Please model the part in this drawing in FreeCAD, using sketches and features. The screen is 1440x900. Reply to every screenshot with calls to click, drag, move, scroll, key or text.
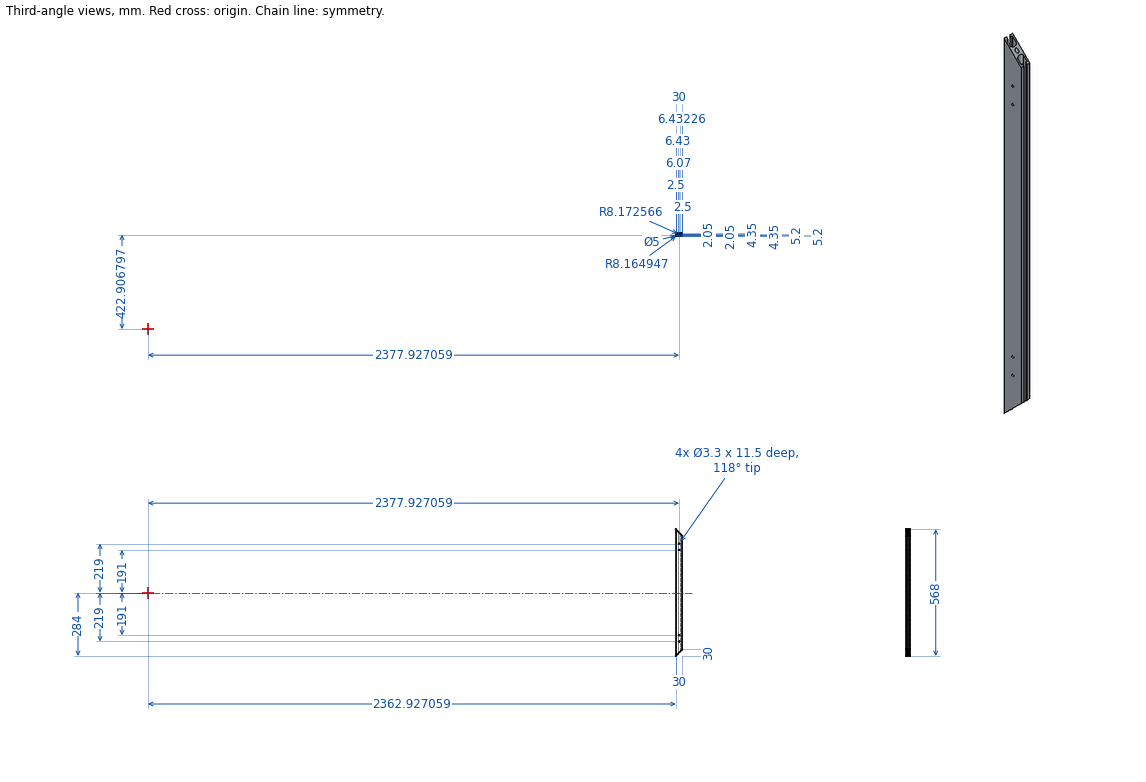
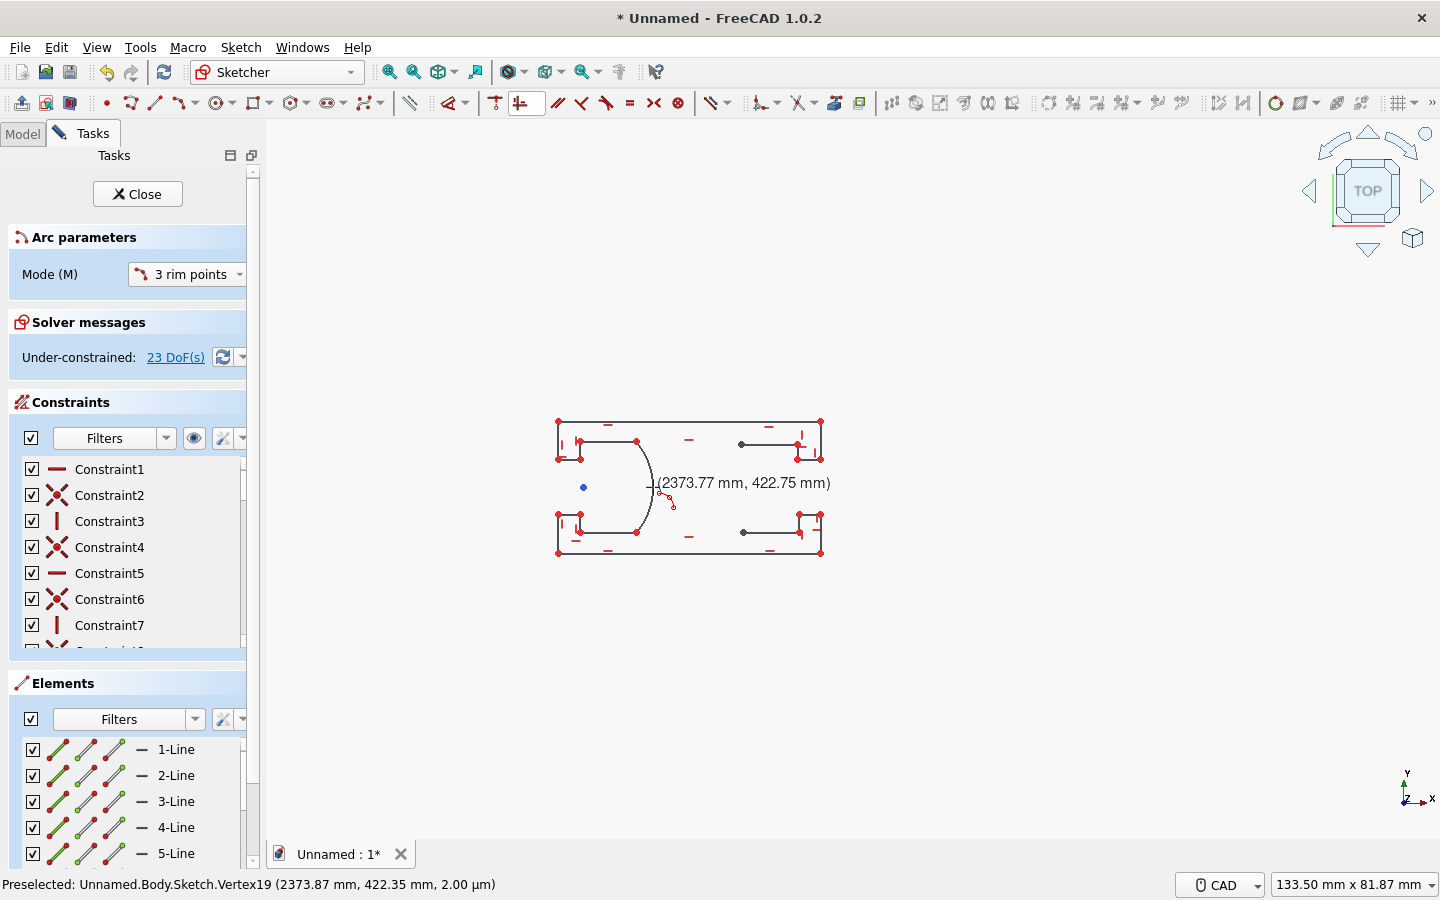
click(743, 533)
click(742, 445)
click(726, 487)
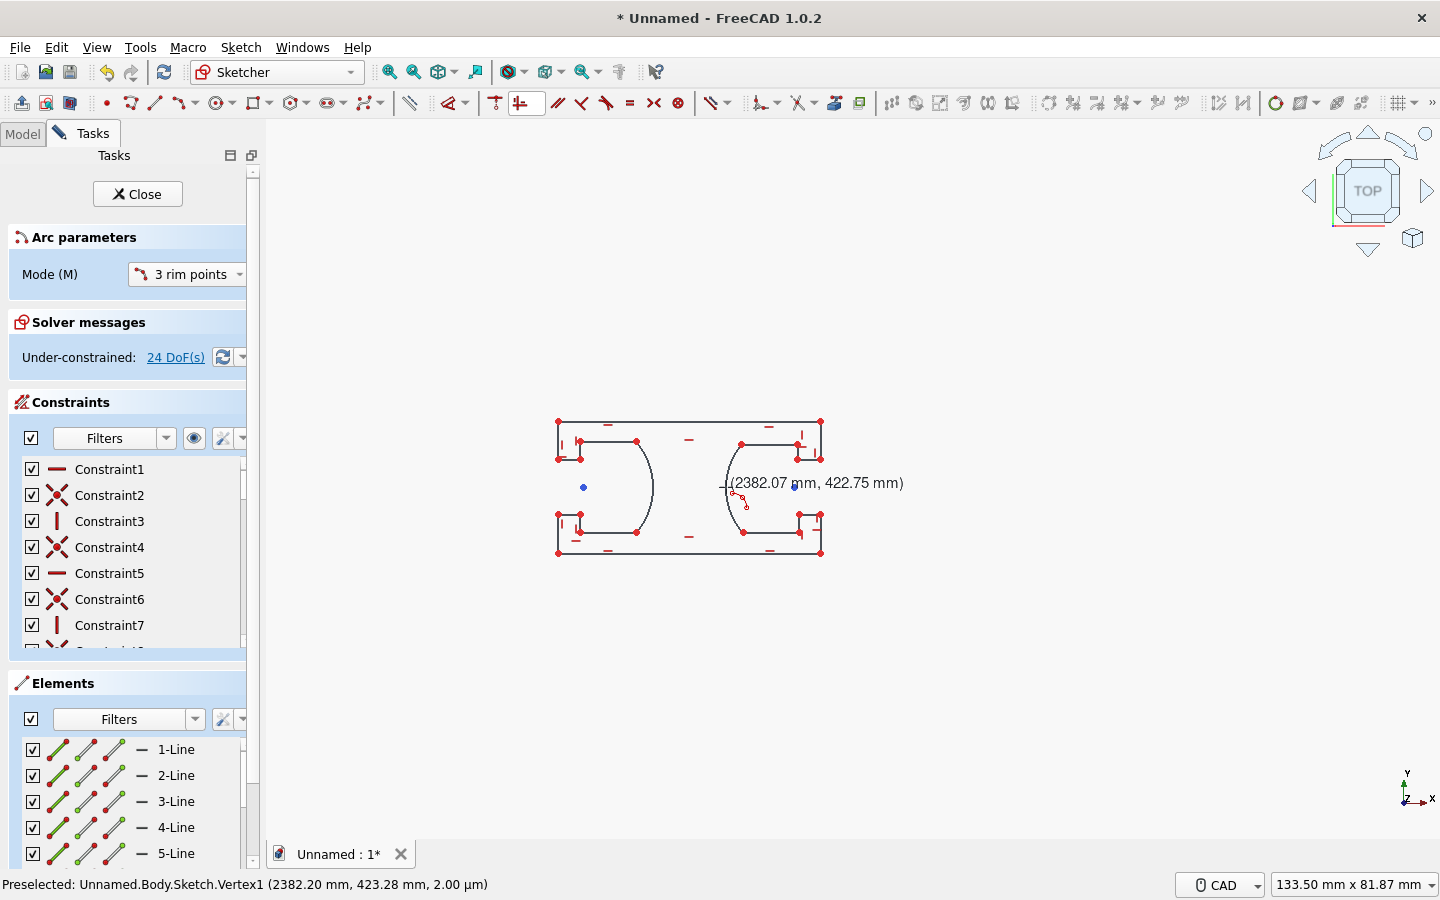
click(216, 104)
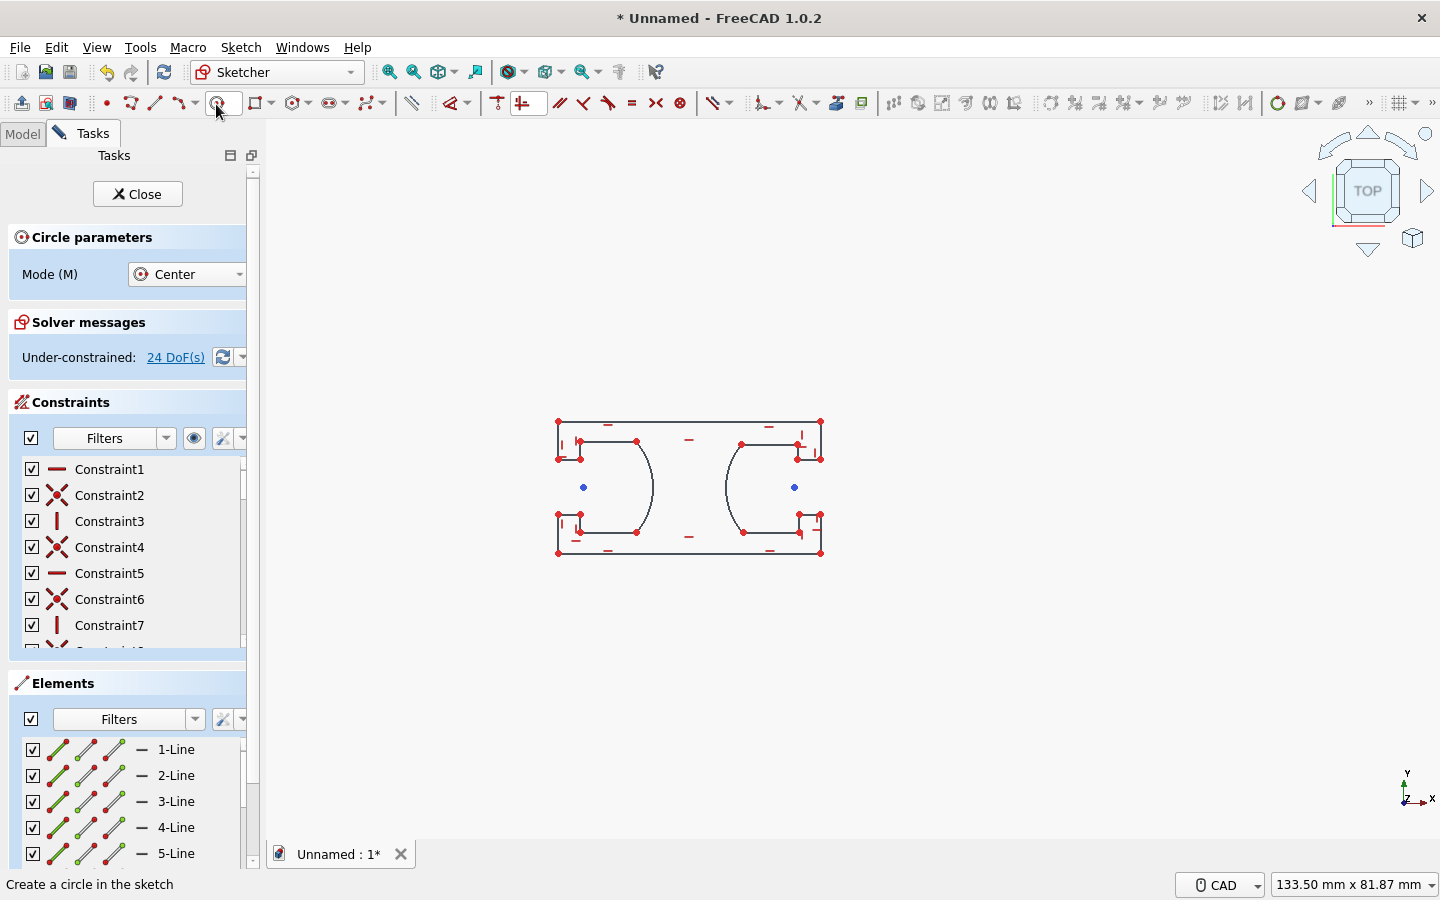
click(690, 487)
move(705, 471)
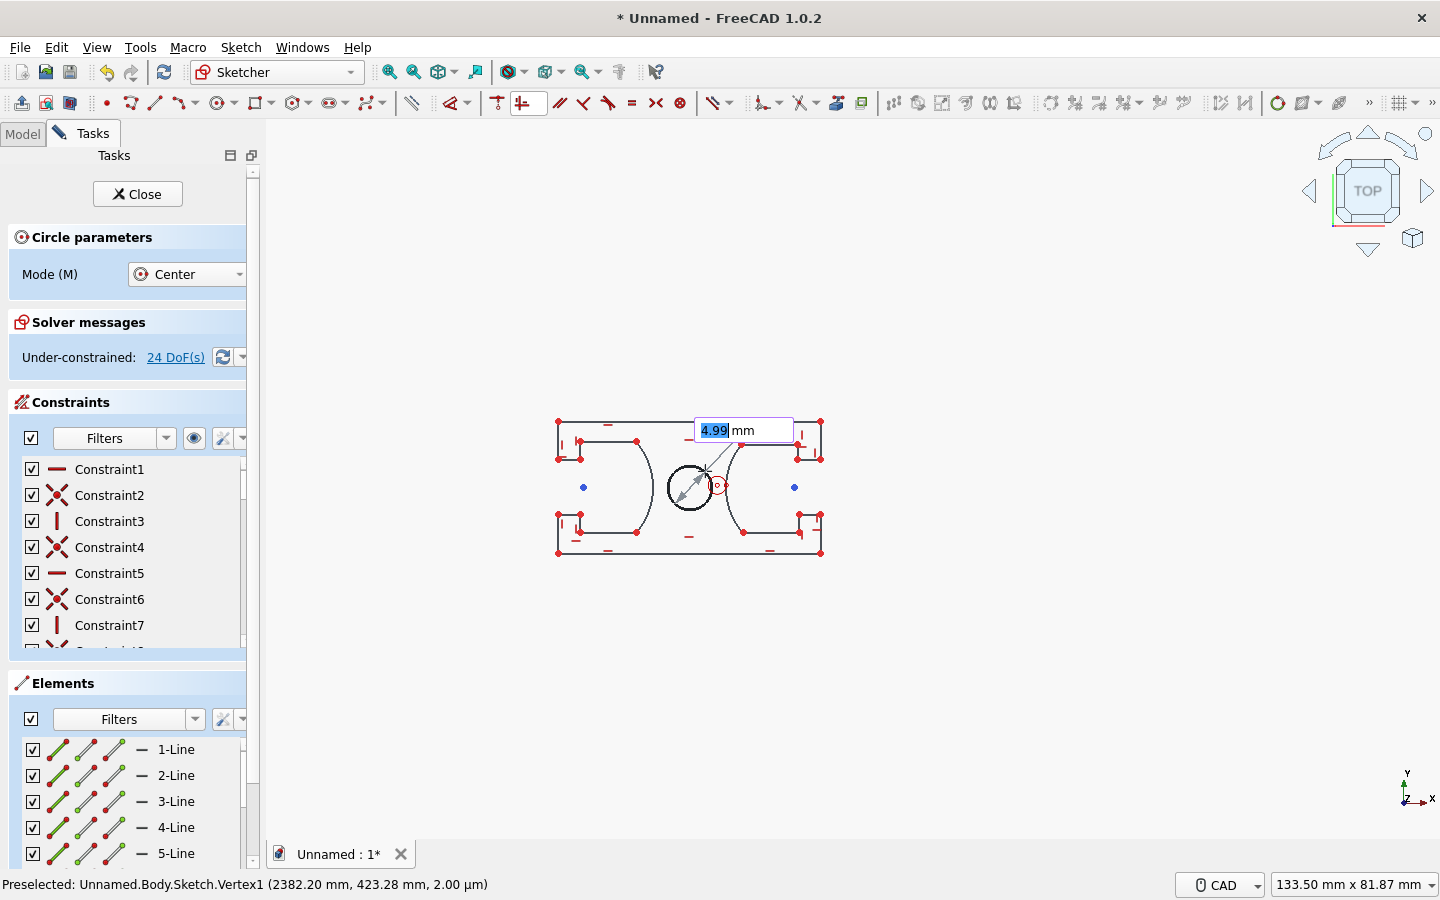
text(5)
key(Return)
key(Escape)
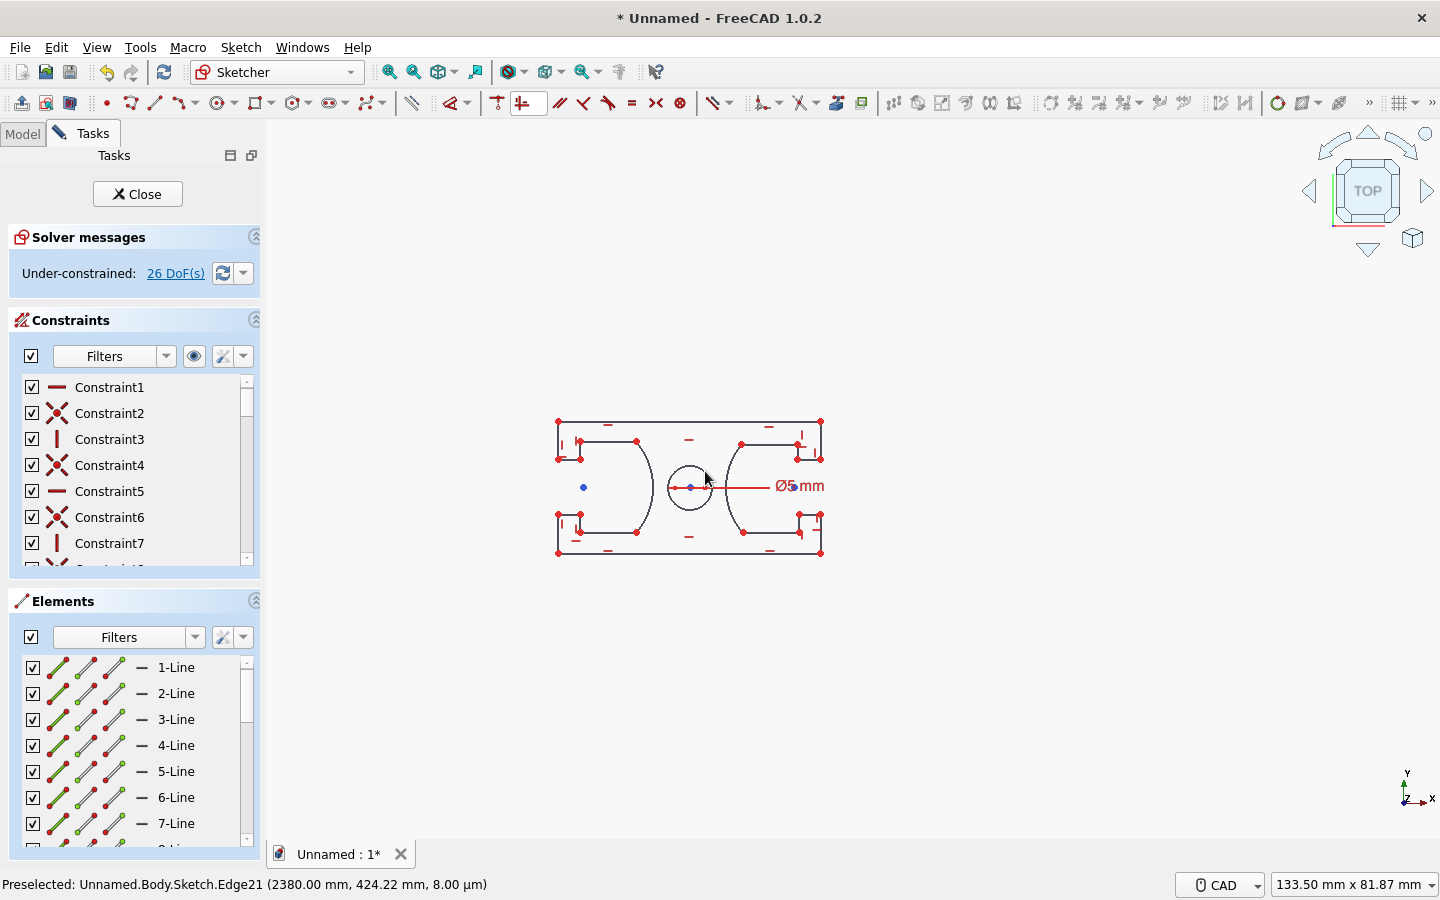
click(450, 104)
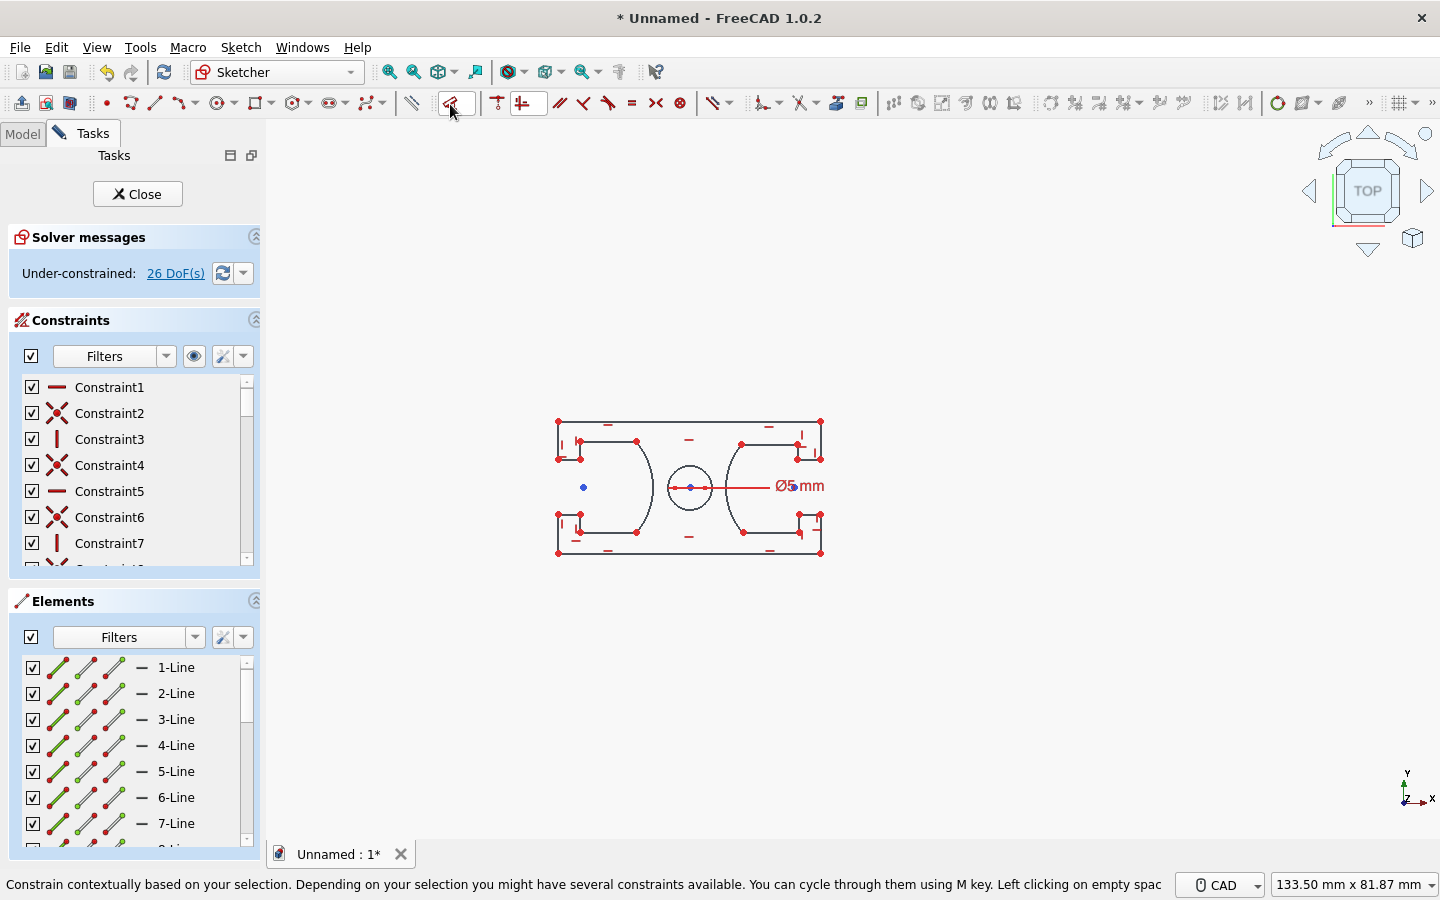
click(650, 507)
click(612, 585)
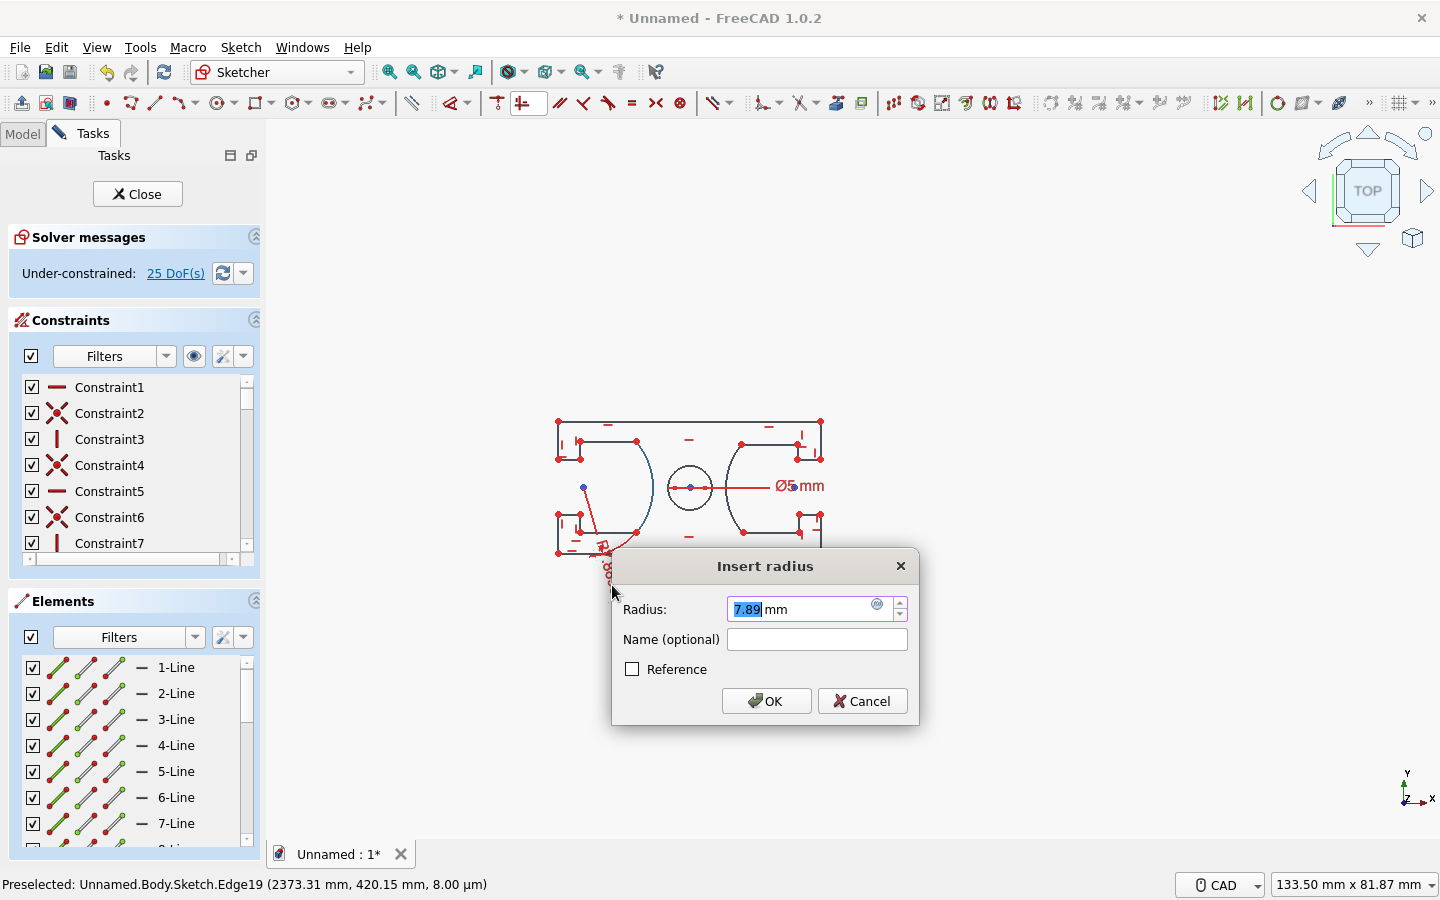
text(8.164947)
key(Return)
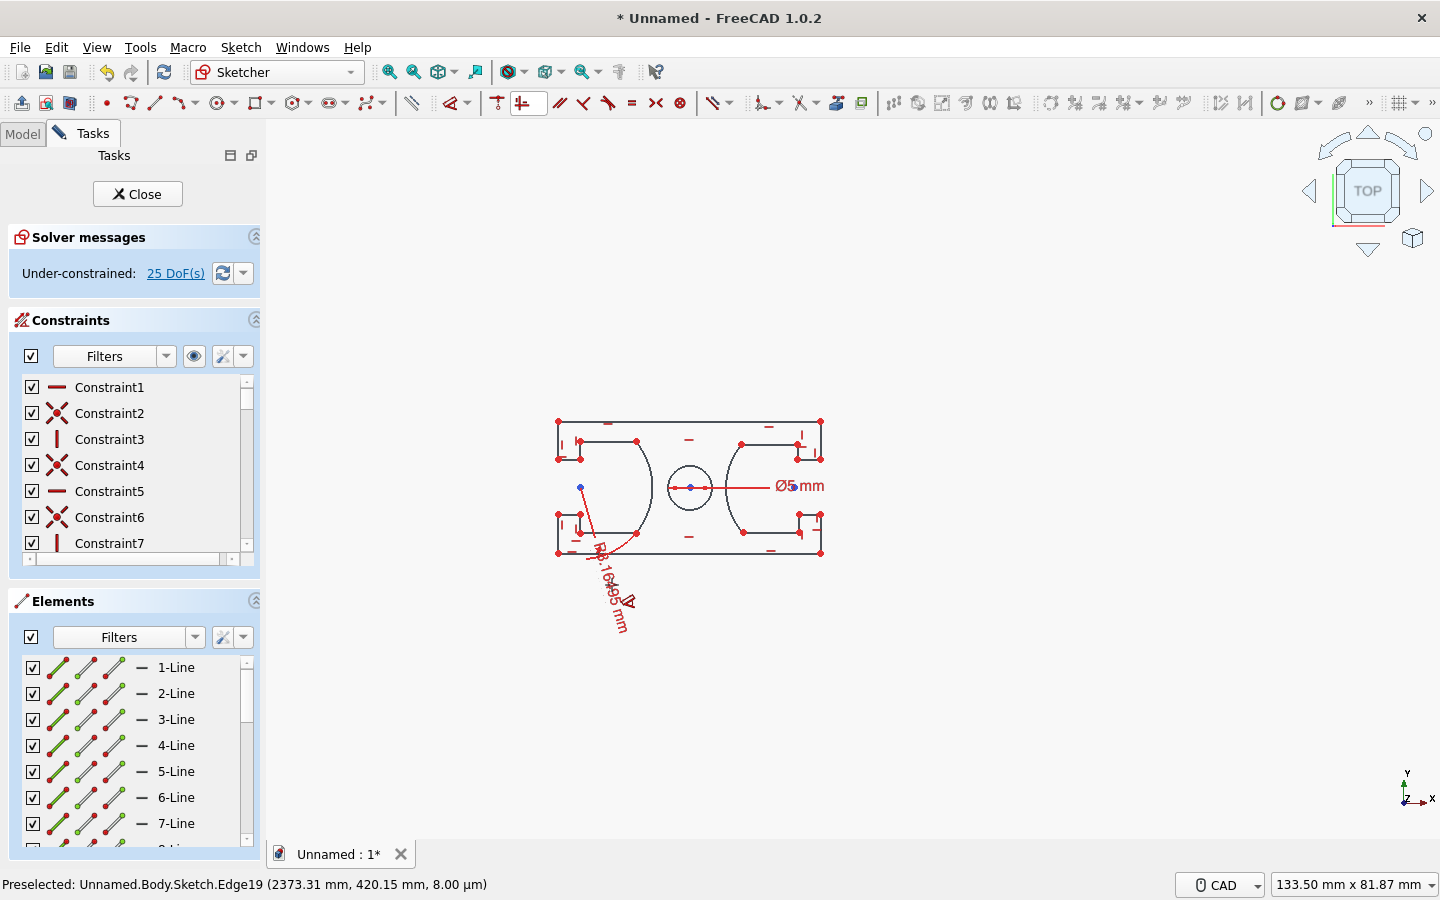
click(728, 470)
click(764, 392)